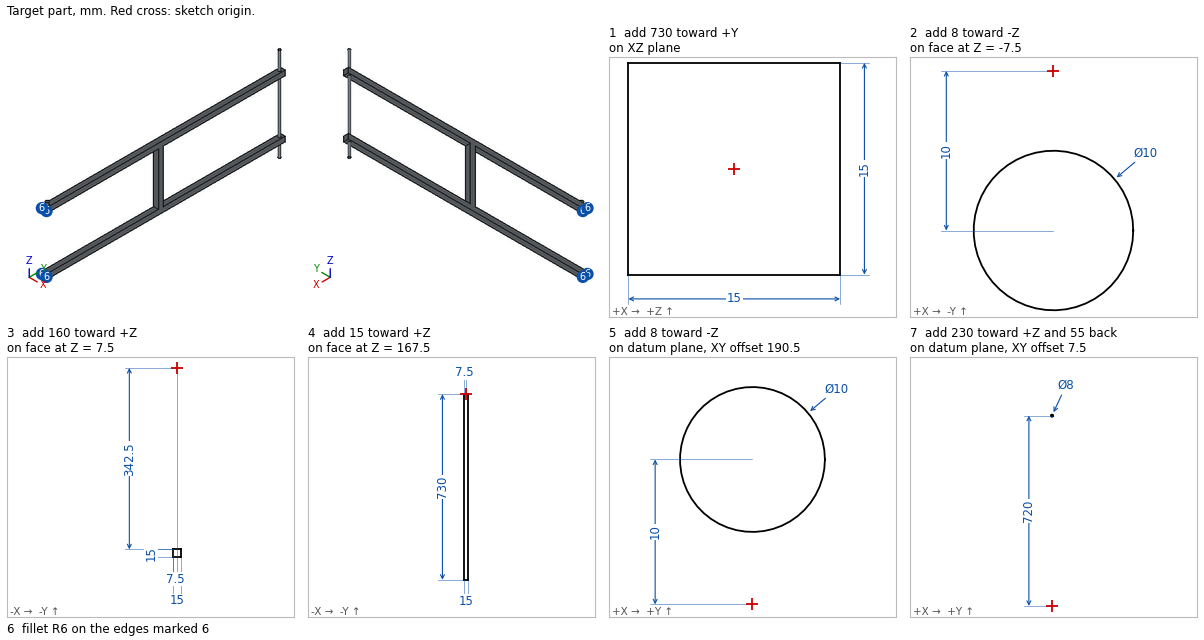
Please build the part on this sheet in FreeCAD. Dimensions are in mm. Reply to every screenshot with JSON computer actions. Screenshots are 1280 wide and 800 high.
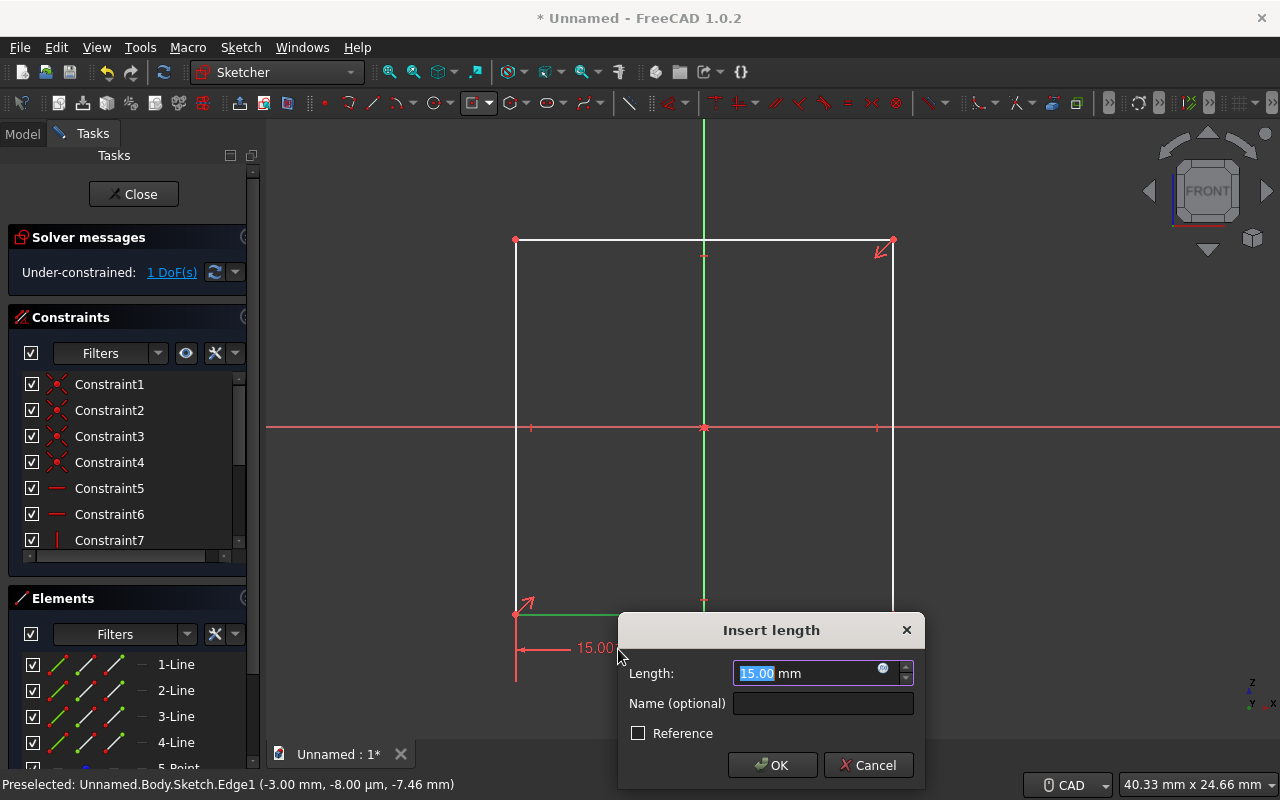
{"action": "type", "text": "15"}
{"action": "key", "text": "Return"}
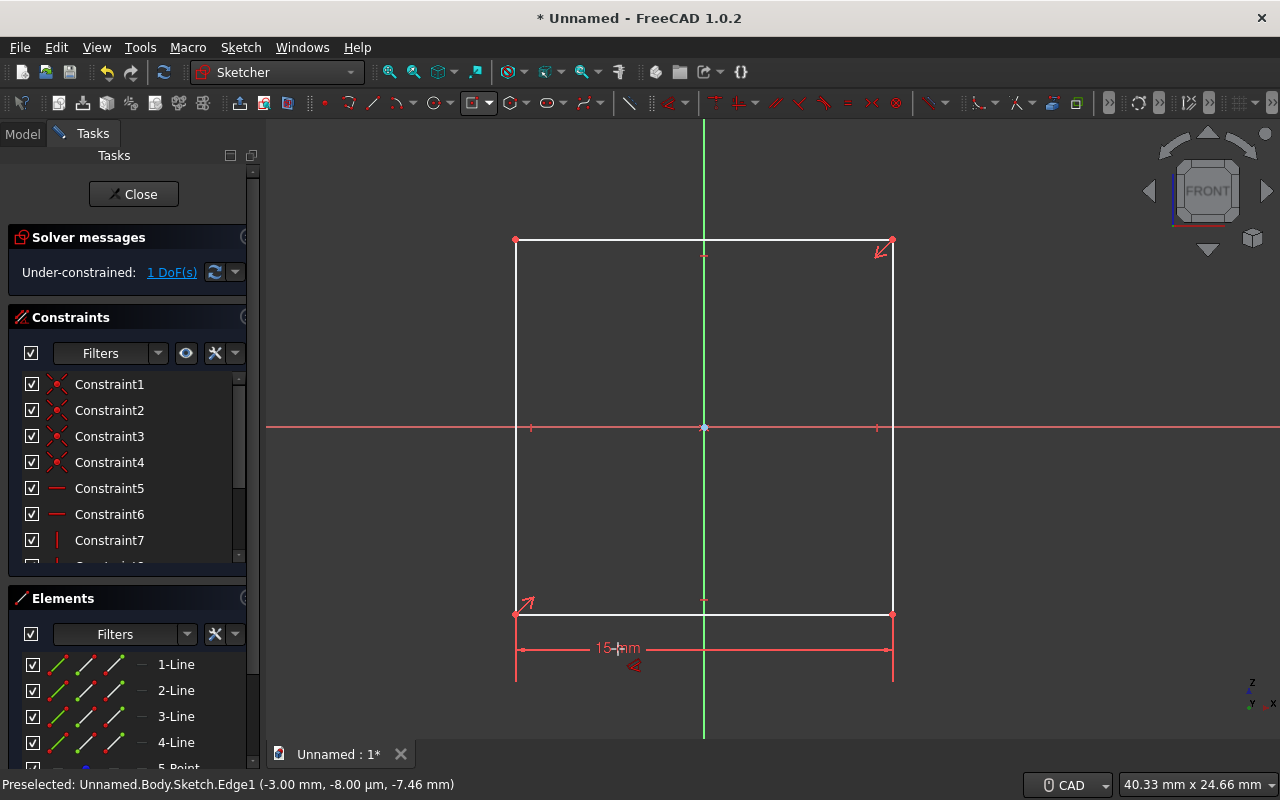
{"action": "left_click", "coordinate": [893, 502]}
{"action": "left_click", "coordinate": [927, 341]}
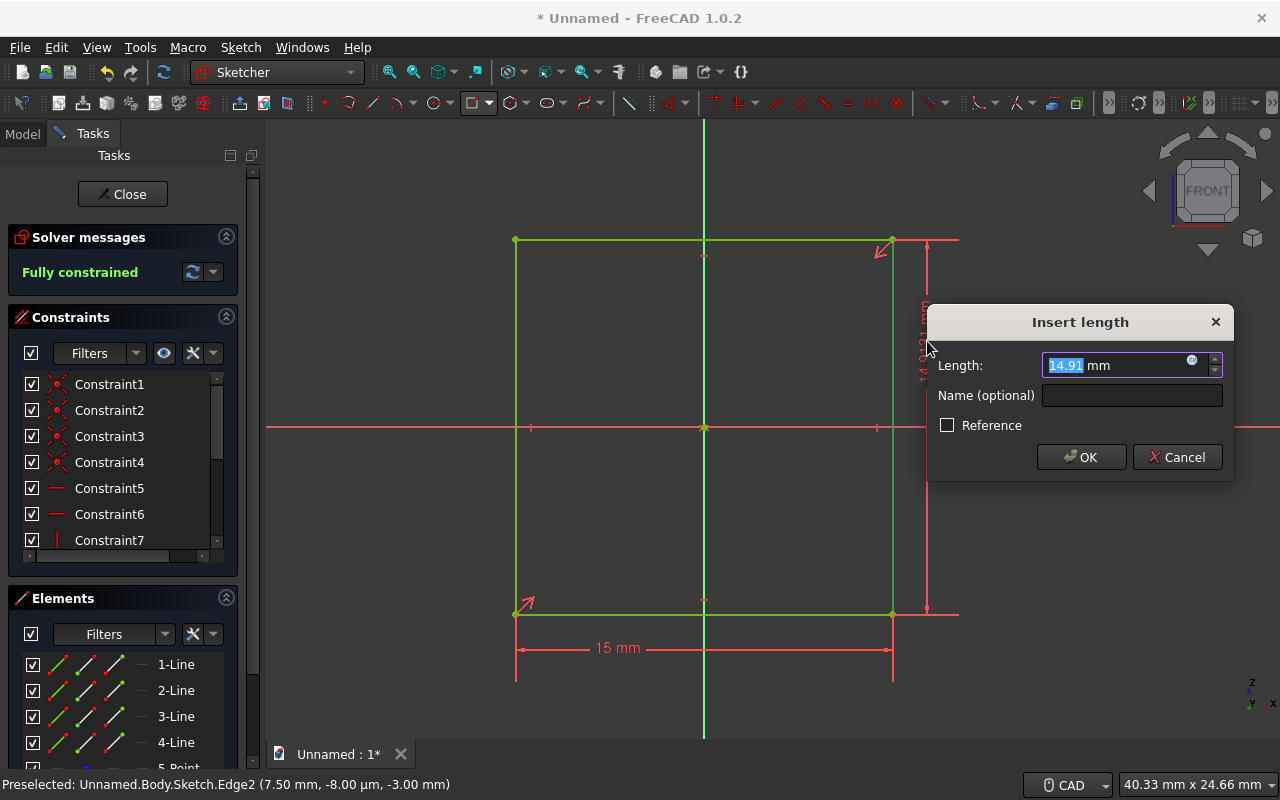
{"action": "type", "text": "15"}
{"action": "key", "text": "Return"}
{"action": "key", "text": "Escape"}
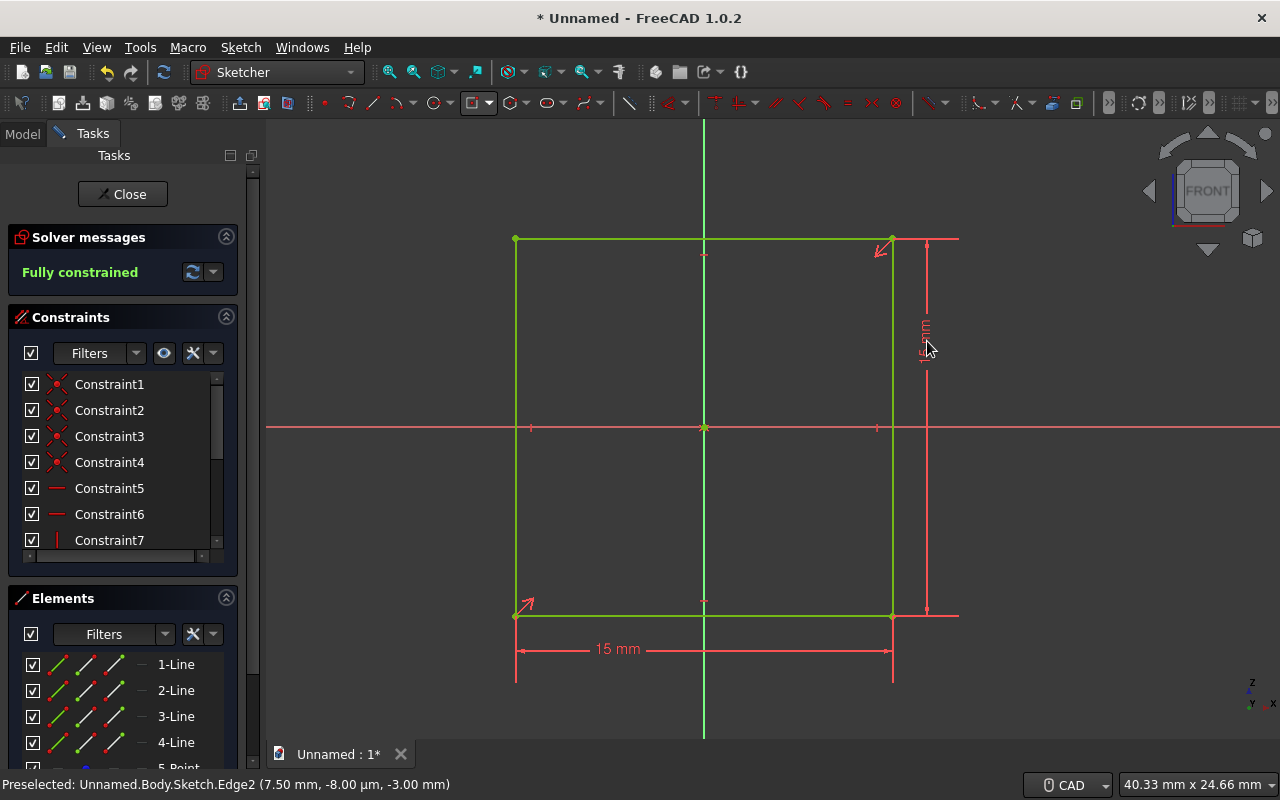
{"action": "left_click", "coordinate": [123, 194]}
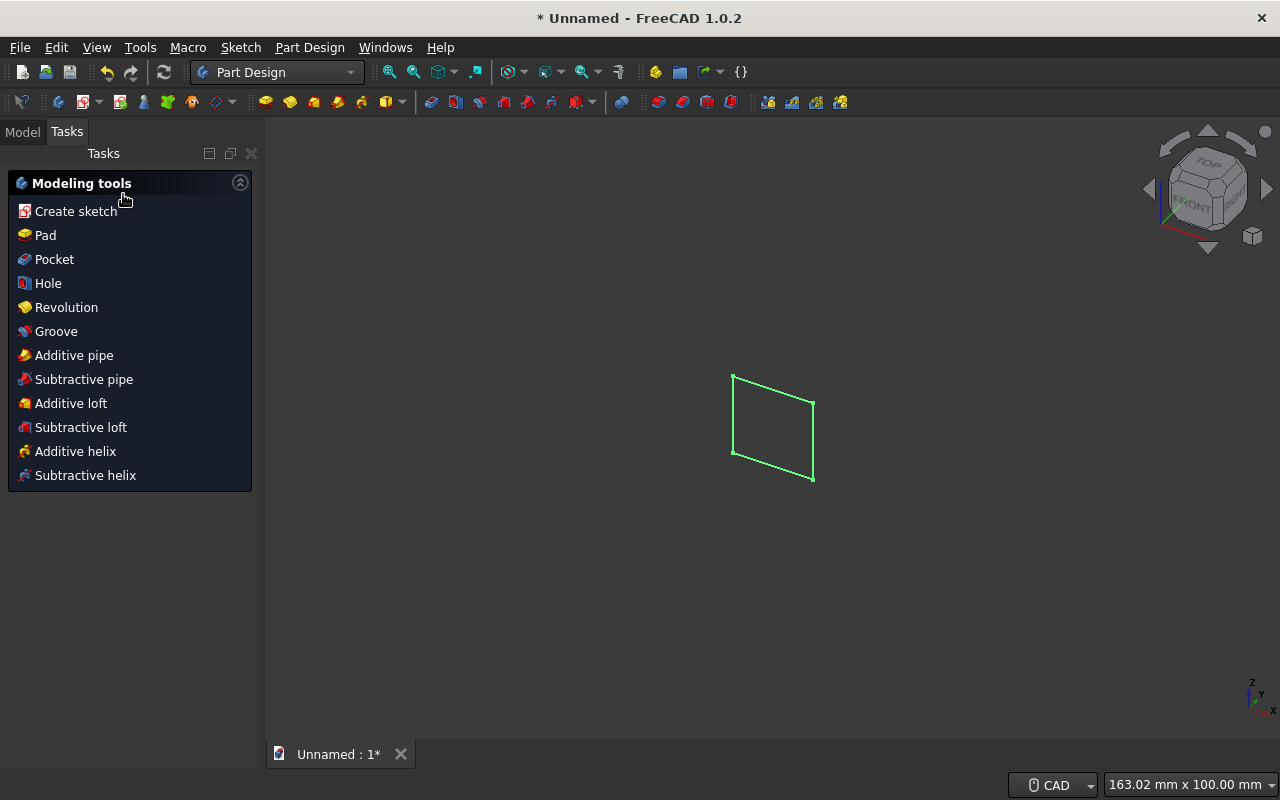
{"action": "left_click", "coordinate": [266, 102]}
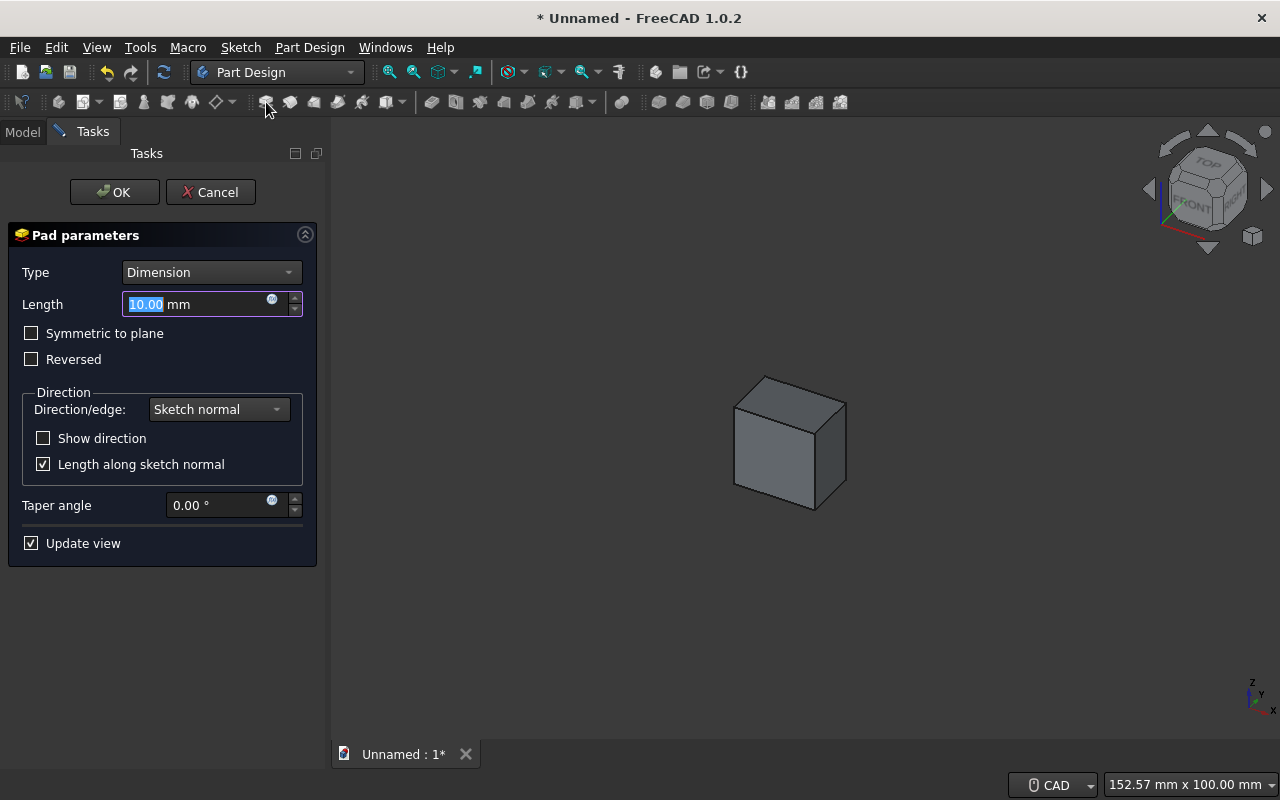
{"action": "type", "text": "730"}
{"action": "key", "text": "Tab"}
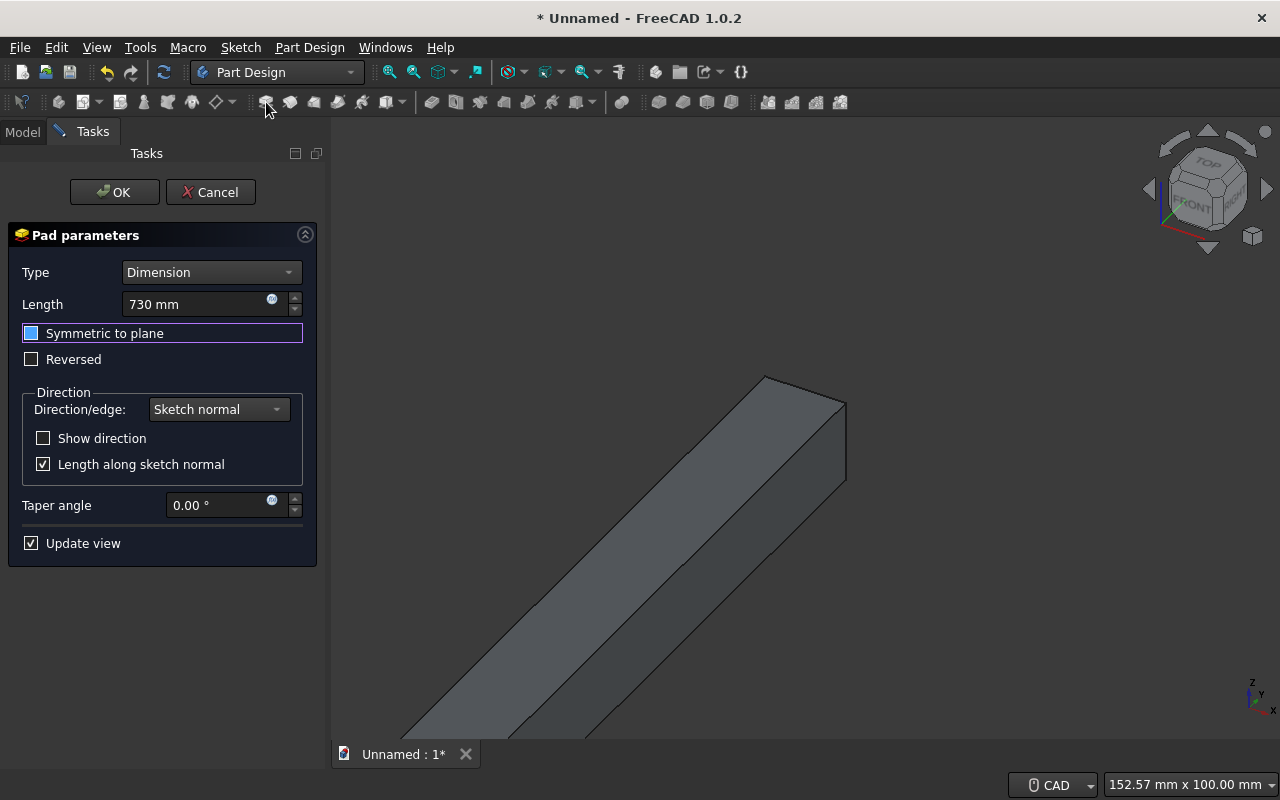
{"action": "left_click", "coordinate": [30, 359]}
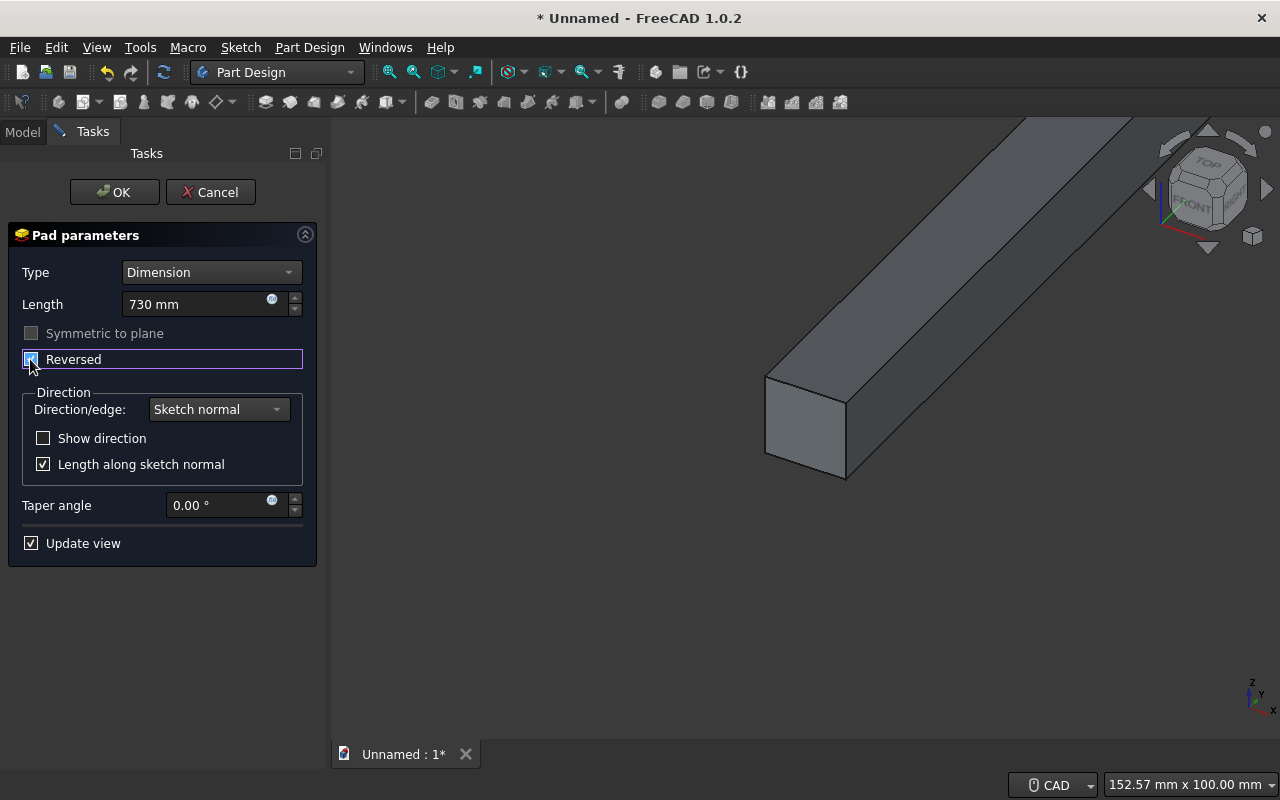
{"action": "left_click", "coordinate": [115, 192]}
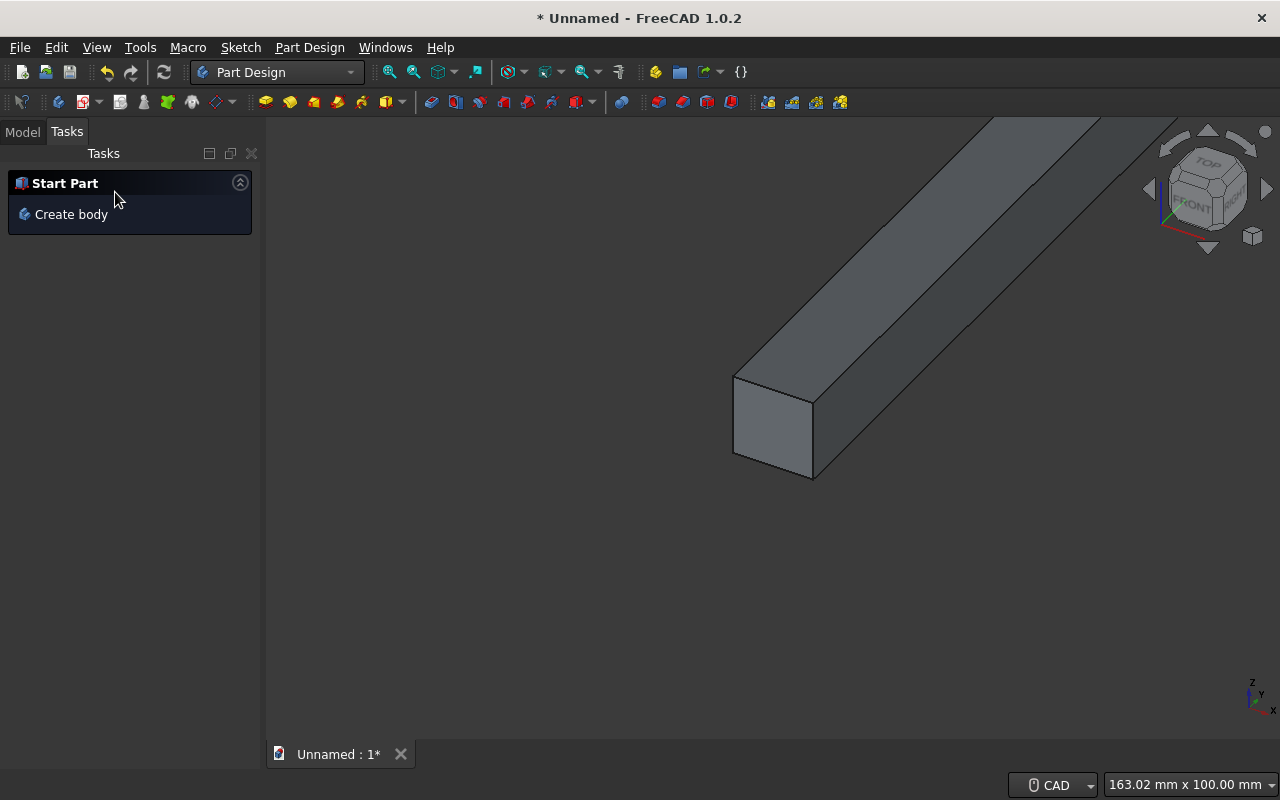
{"action": "left_click", "coordinate": [390, 72]}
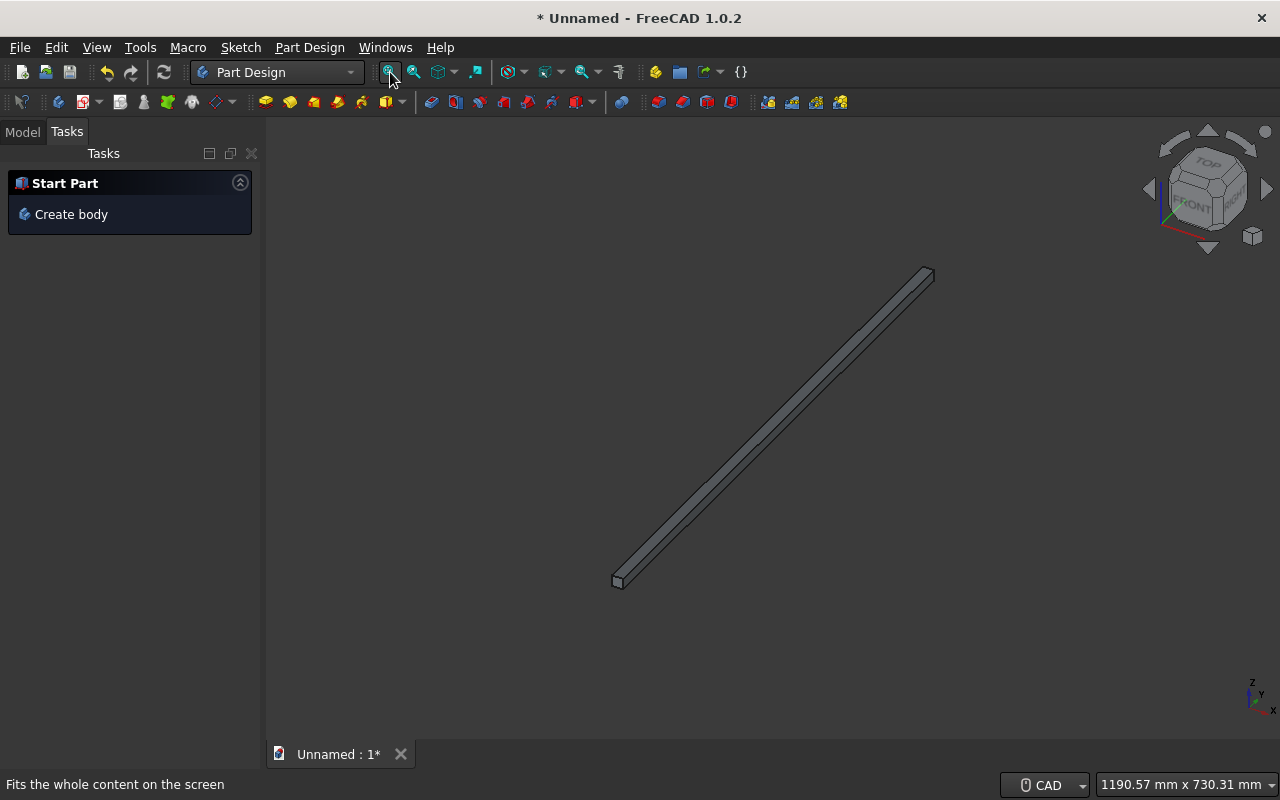
{"action": "key", "text": "5"}